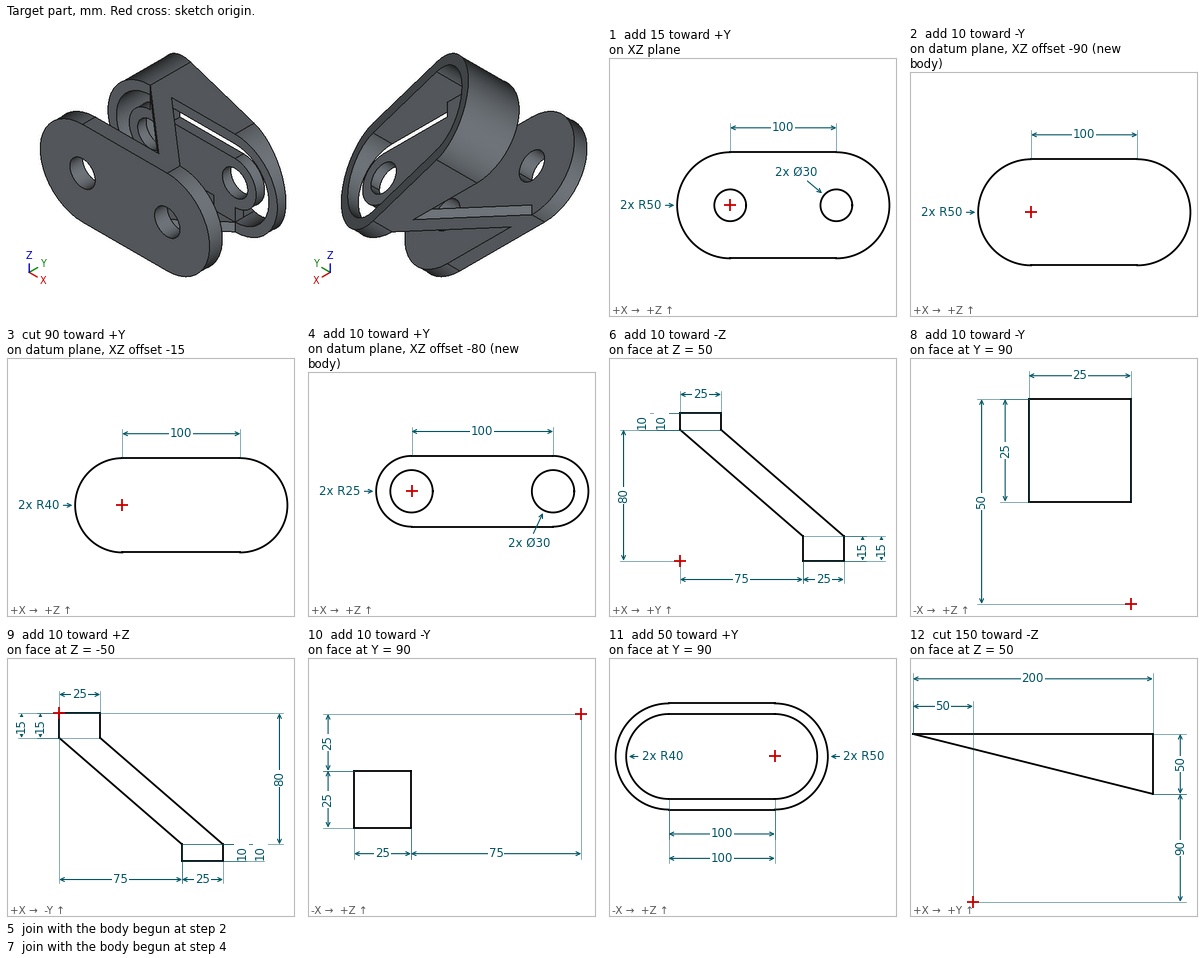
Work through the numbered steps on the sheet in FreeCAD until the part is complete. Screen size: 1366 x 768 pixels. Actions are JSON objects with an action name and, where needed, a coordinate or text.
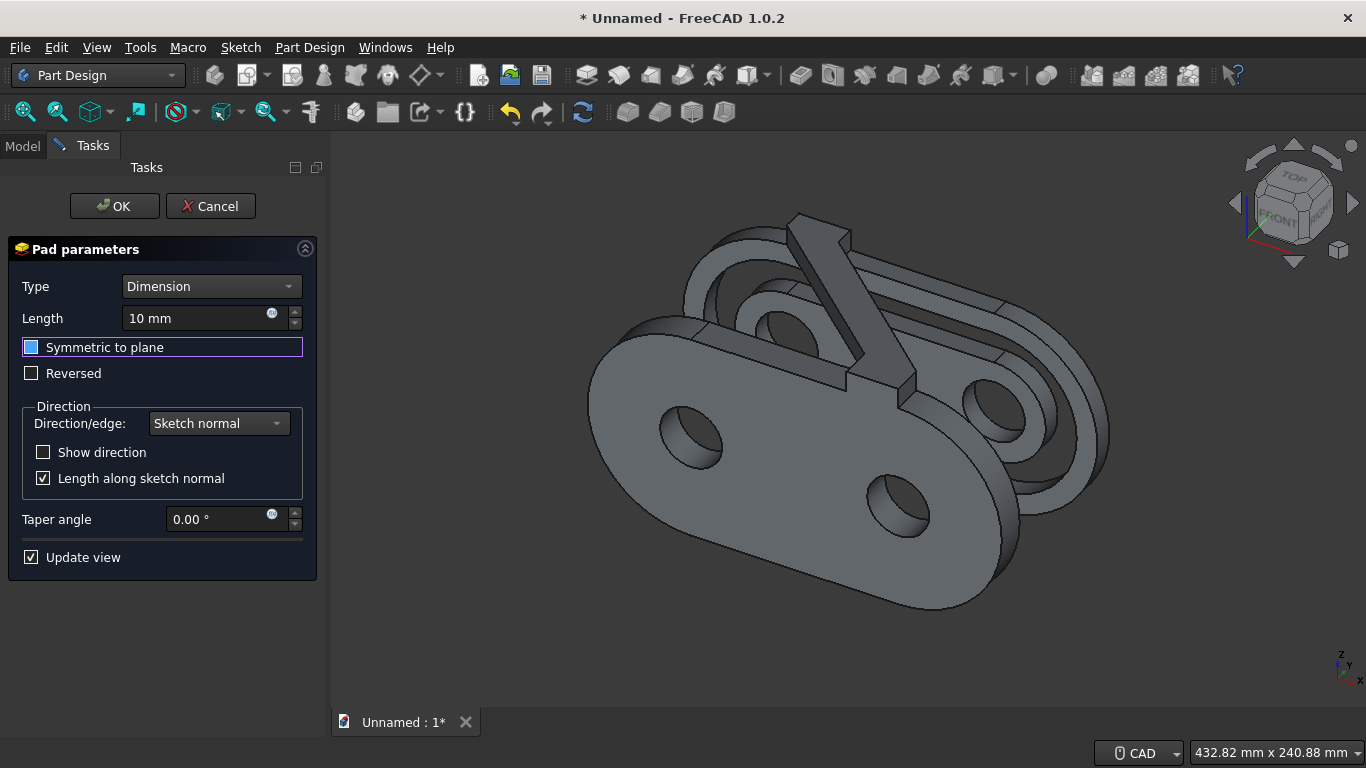
{"action": "left_click", "coordinate": [30, 373]}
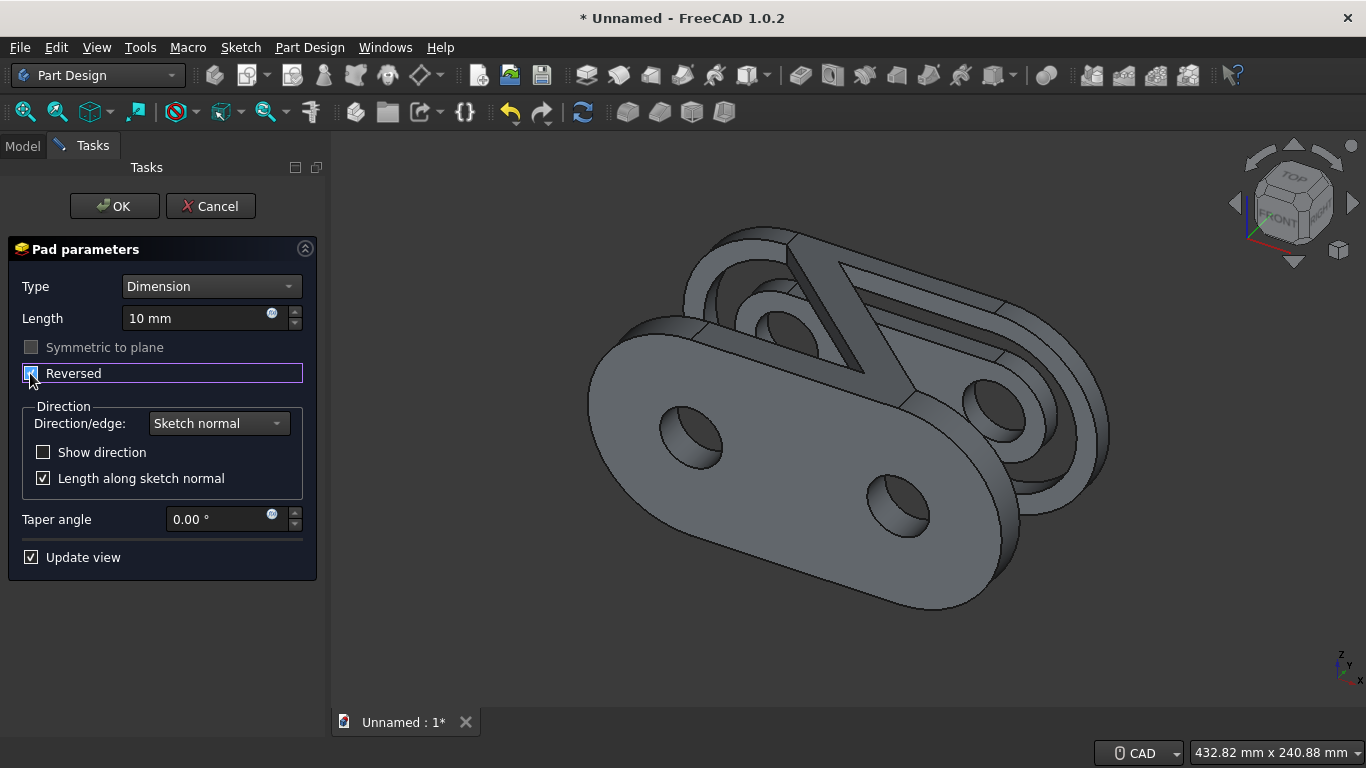
{"action": "left_click", "coordinate": [115, 206]}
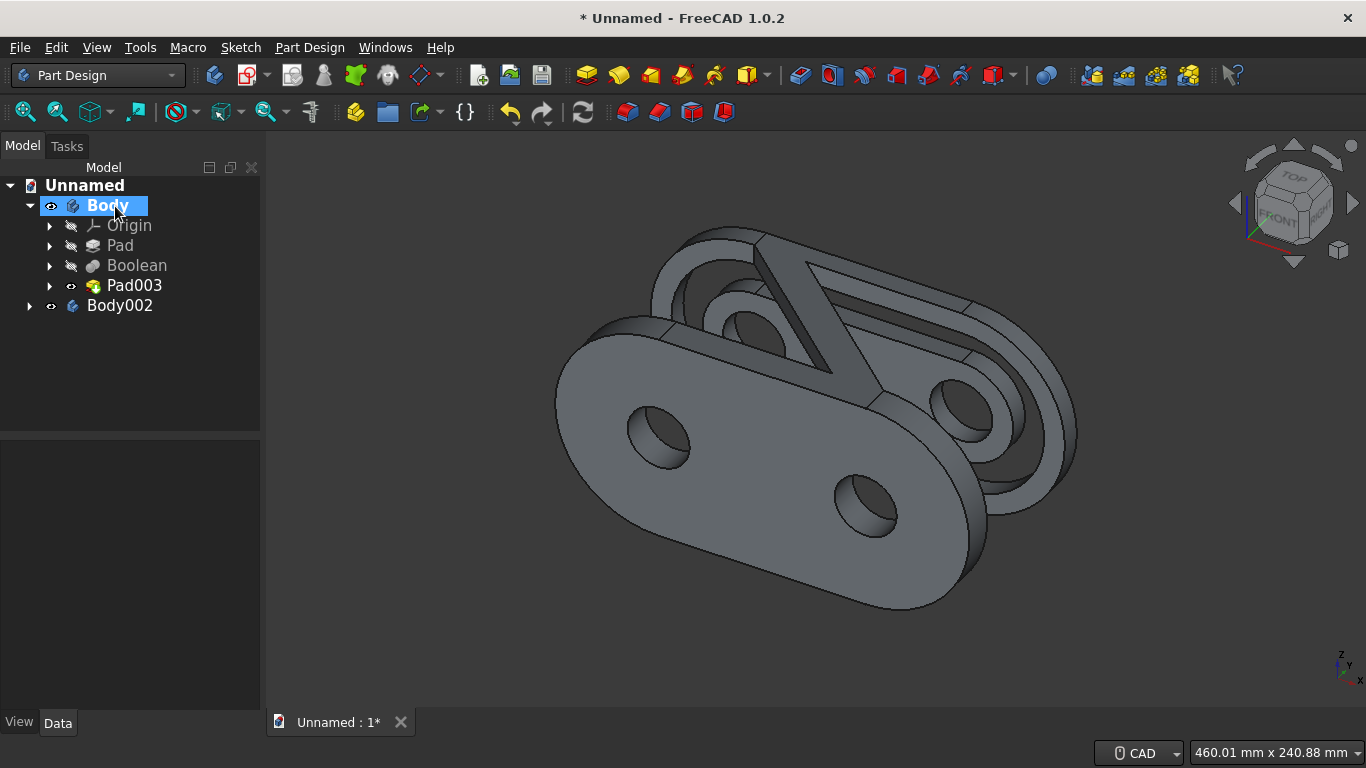
{"action": "left_click", "coordinate": [96, 306]}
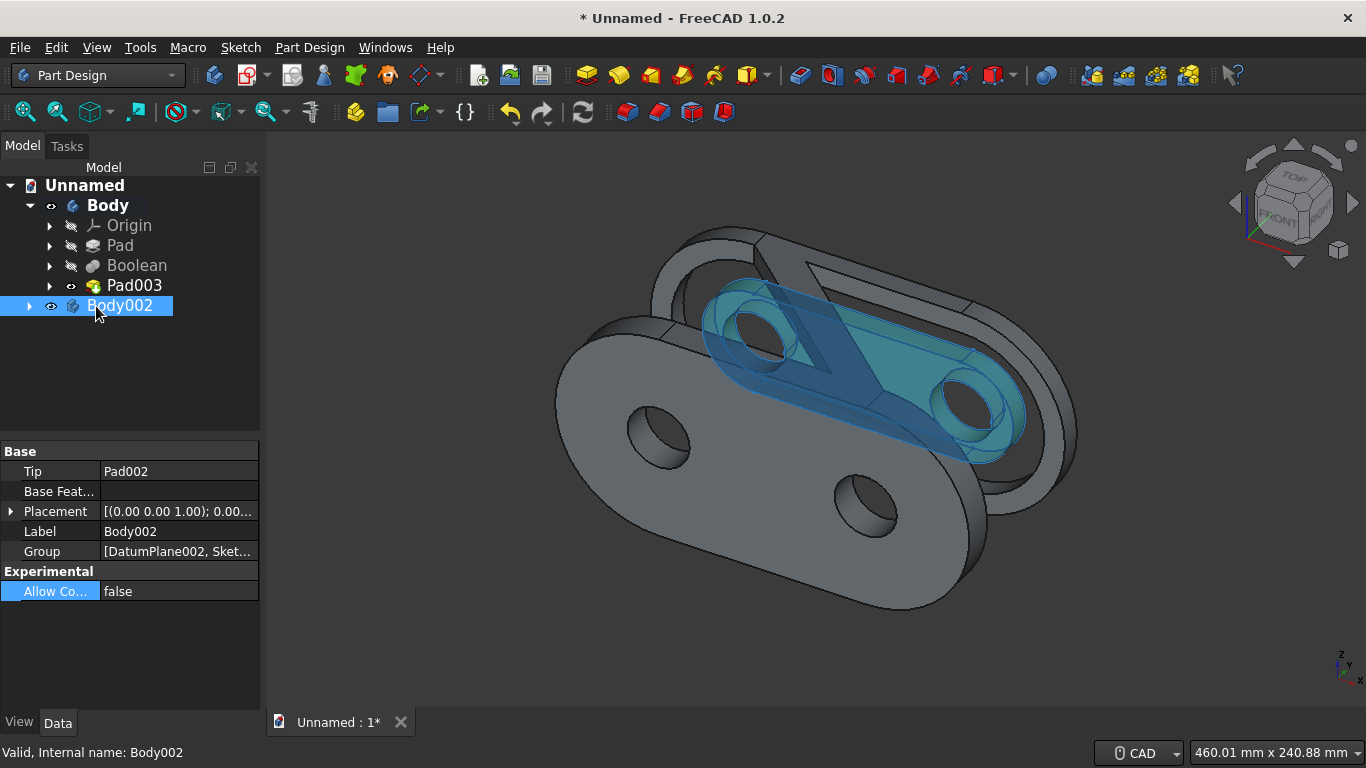
{"action": "left_click", "coordinate": [1048, 76]}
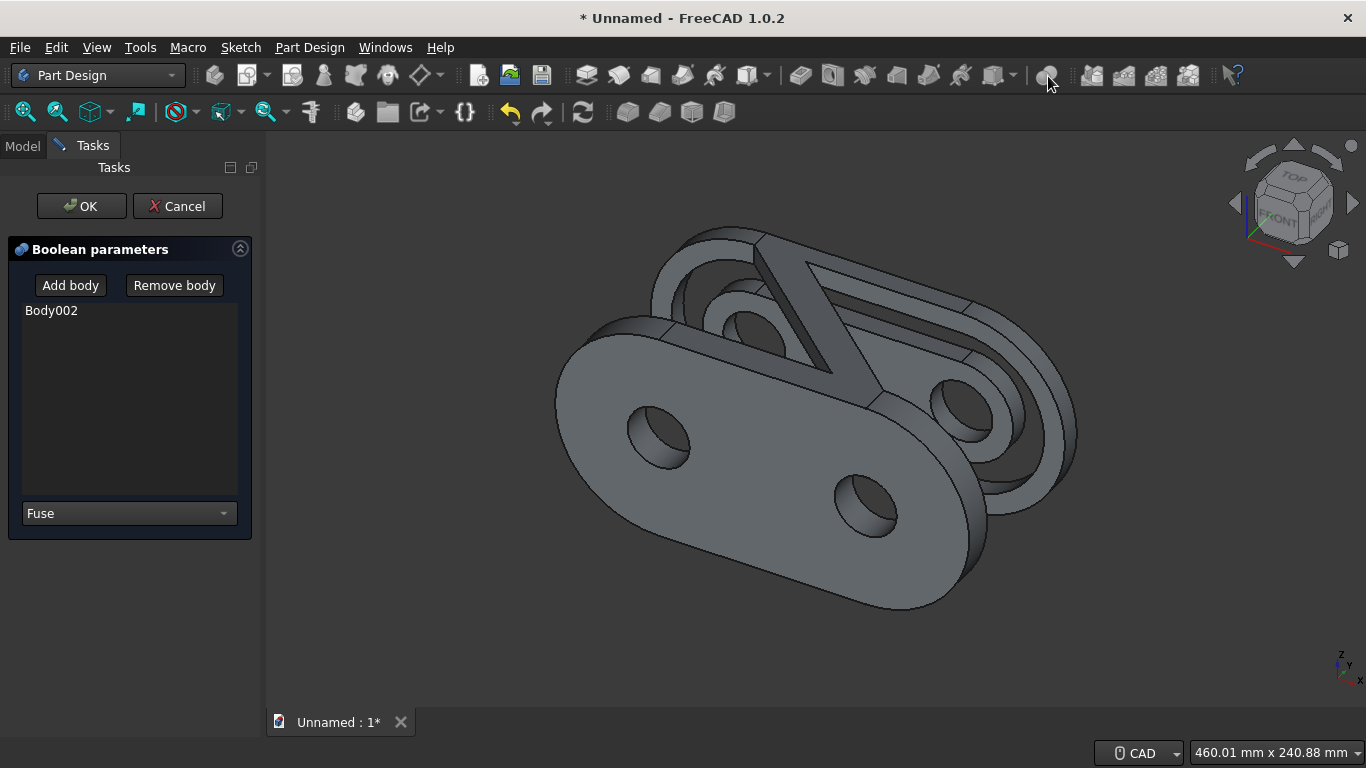
{"action": "left_click", "coordinate": [82, 206]}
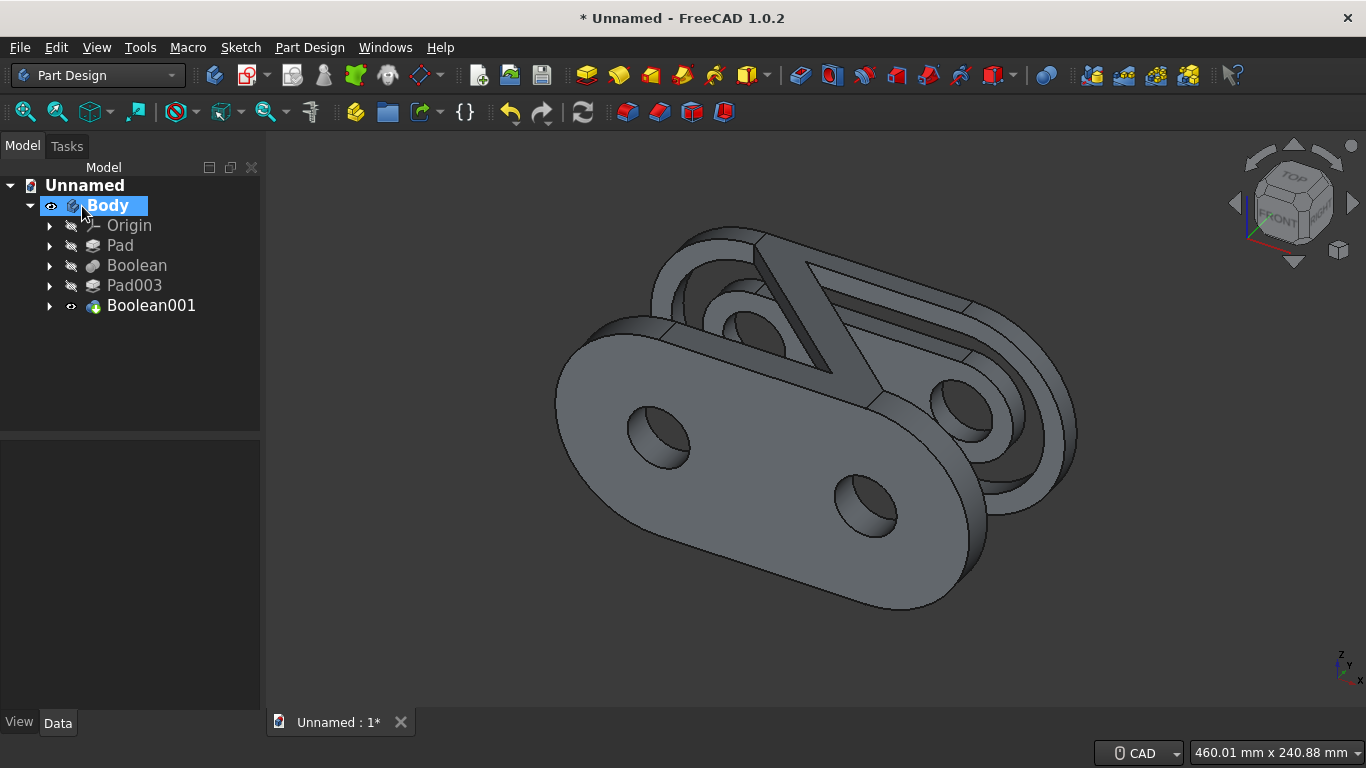
{"action": "key", "text": "4"}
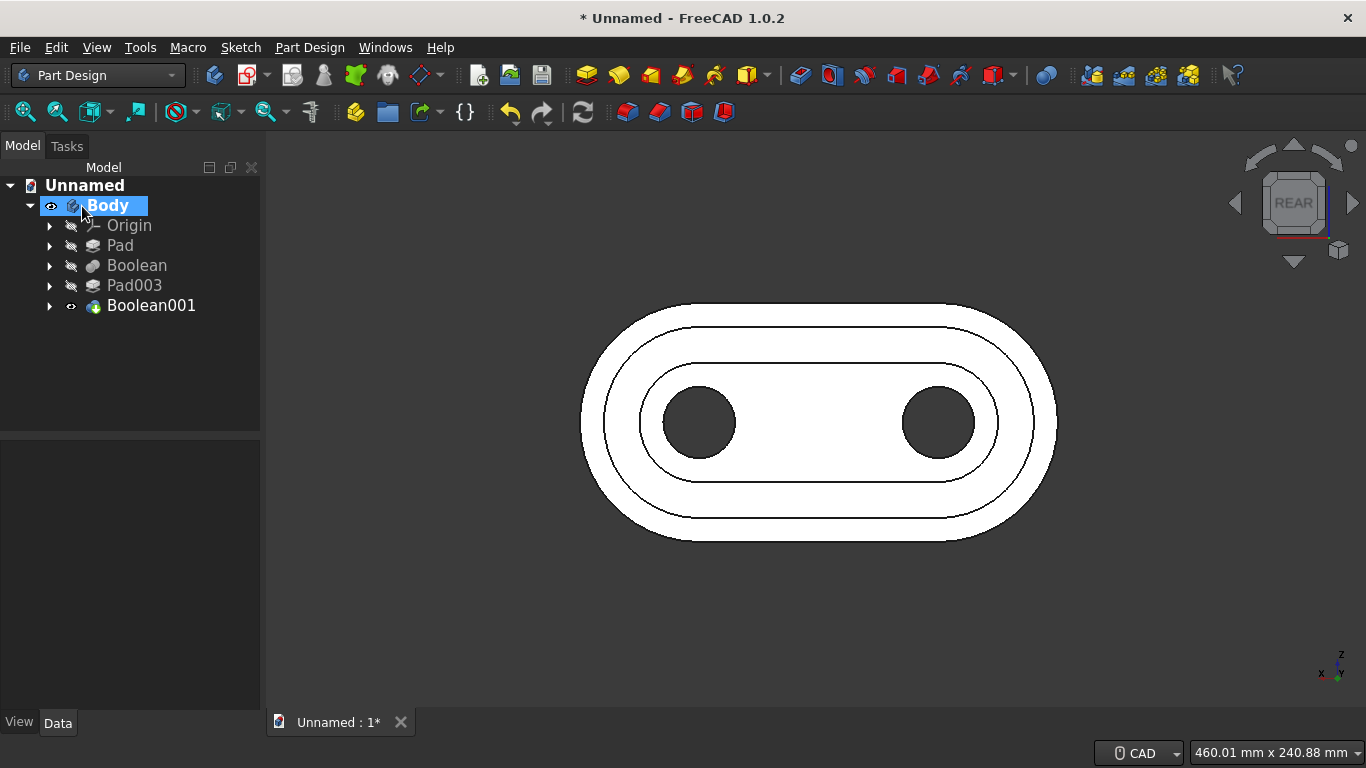
{"action": "left_click", "coordinate": [26, 112]}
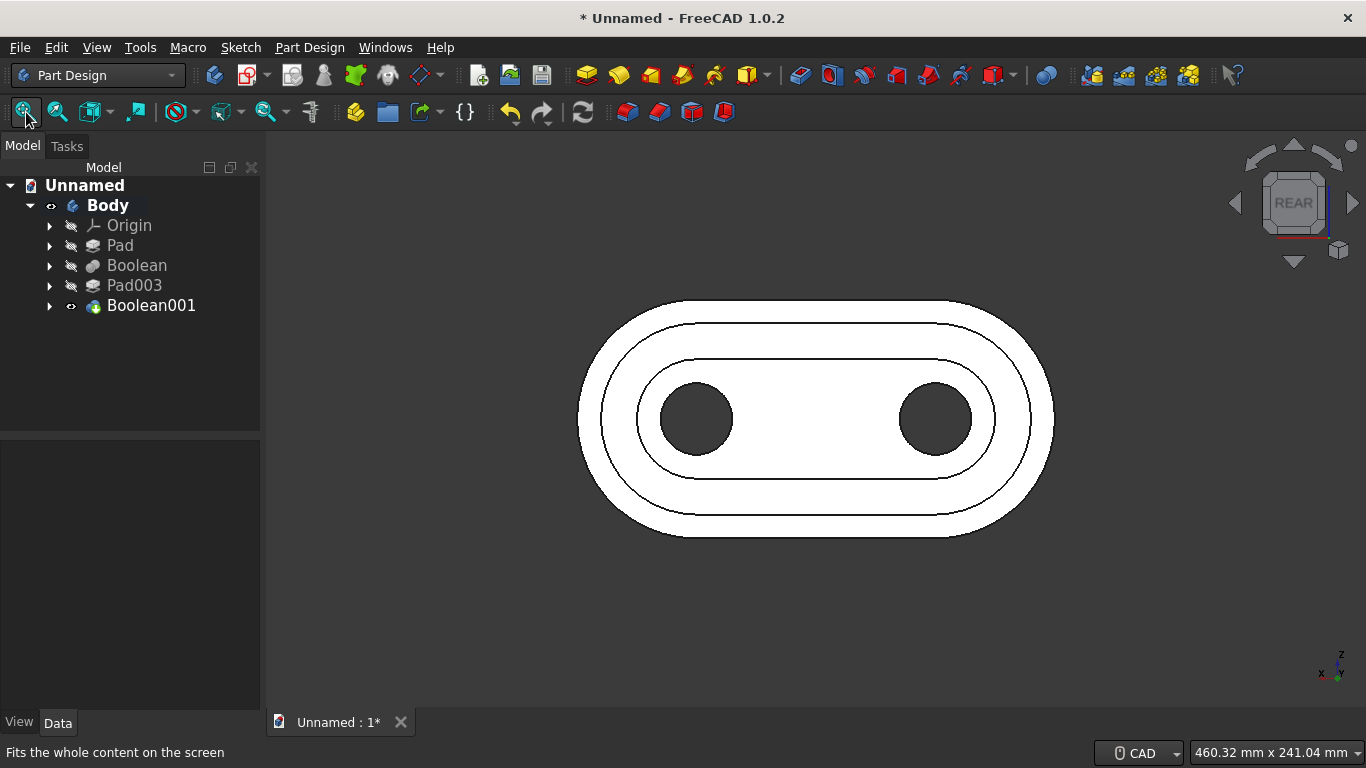
{"action": "left_click", "coordinate": [816, 418]}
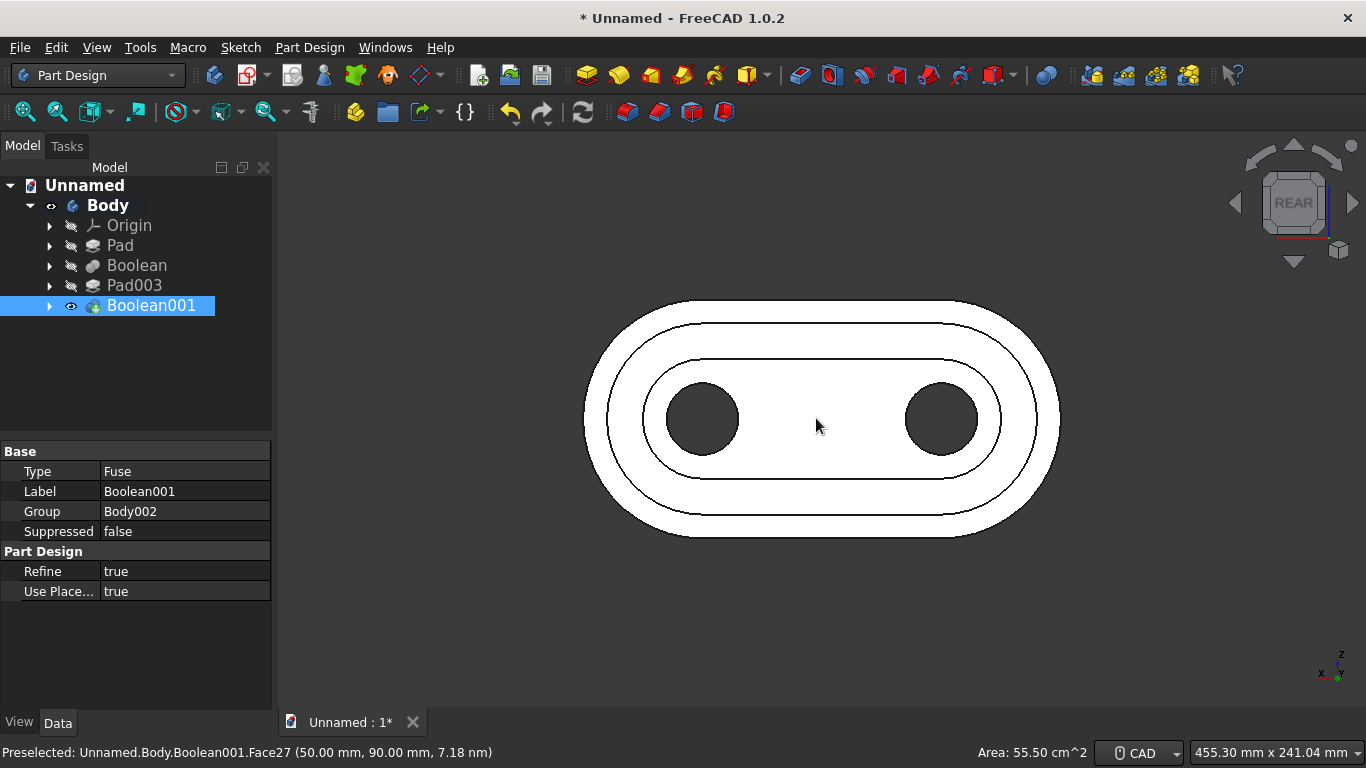
{"action": "left_click", "coordinate": [248, 76]}